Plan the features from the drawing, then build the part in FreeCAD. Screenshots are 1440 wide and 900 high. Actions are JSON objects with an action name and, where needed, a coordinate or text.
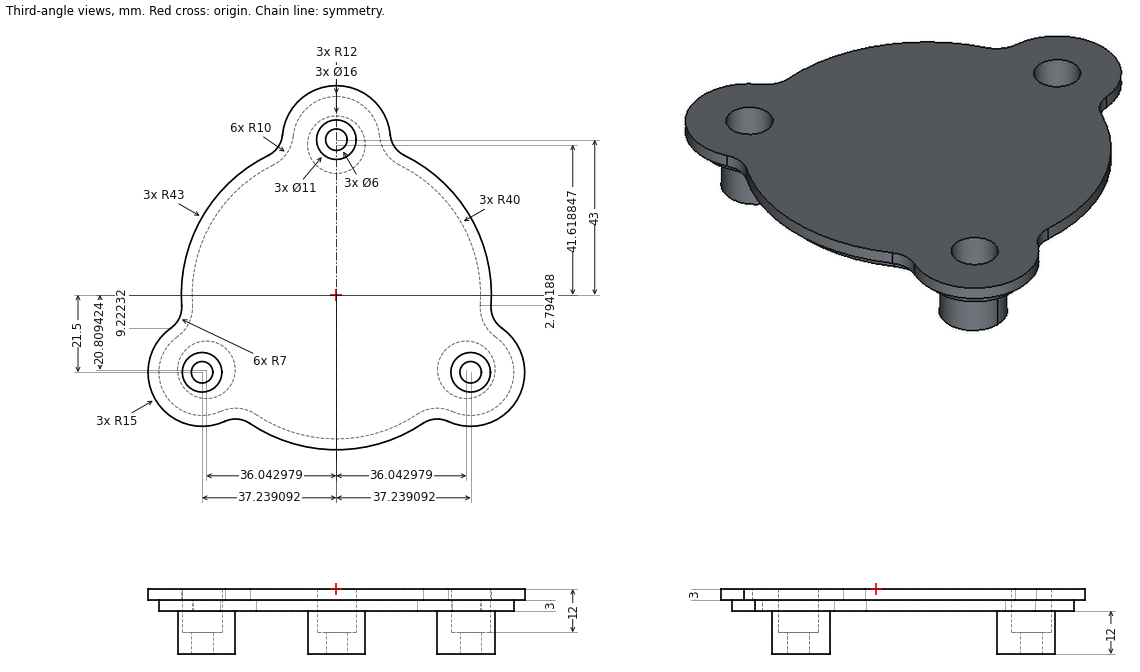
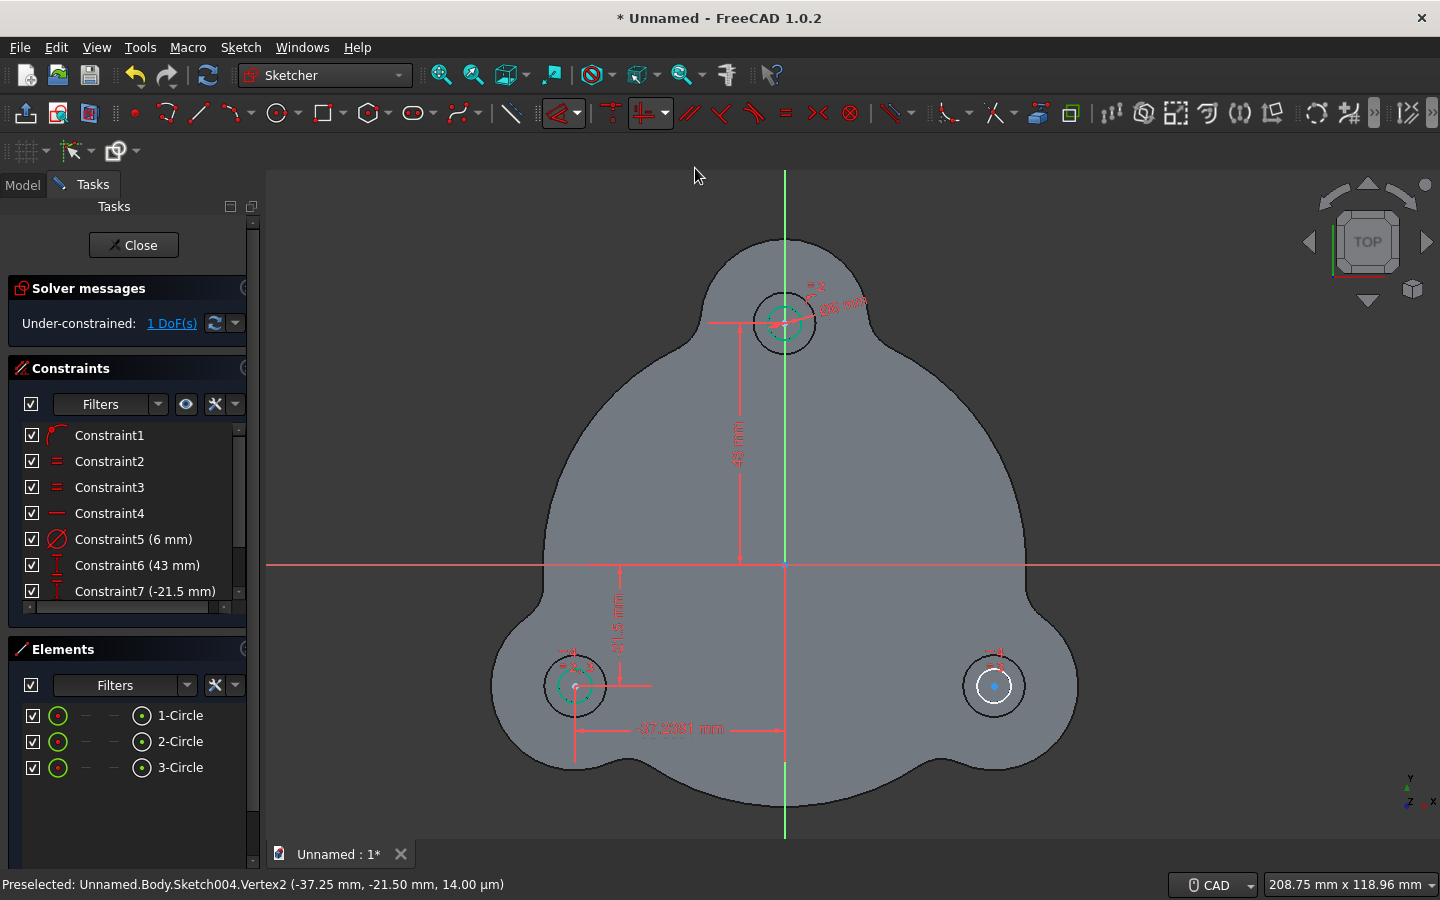
{"action": "left_click", "coordinate": [994, 686]}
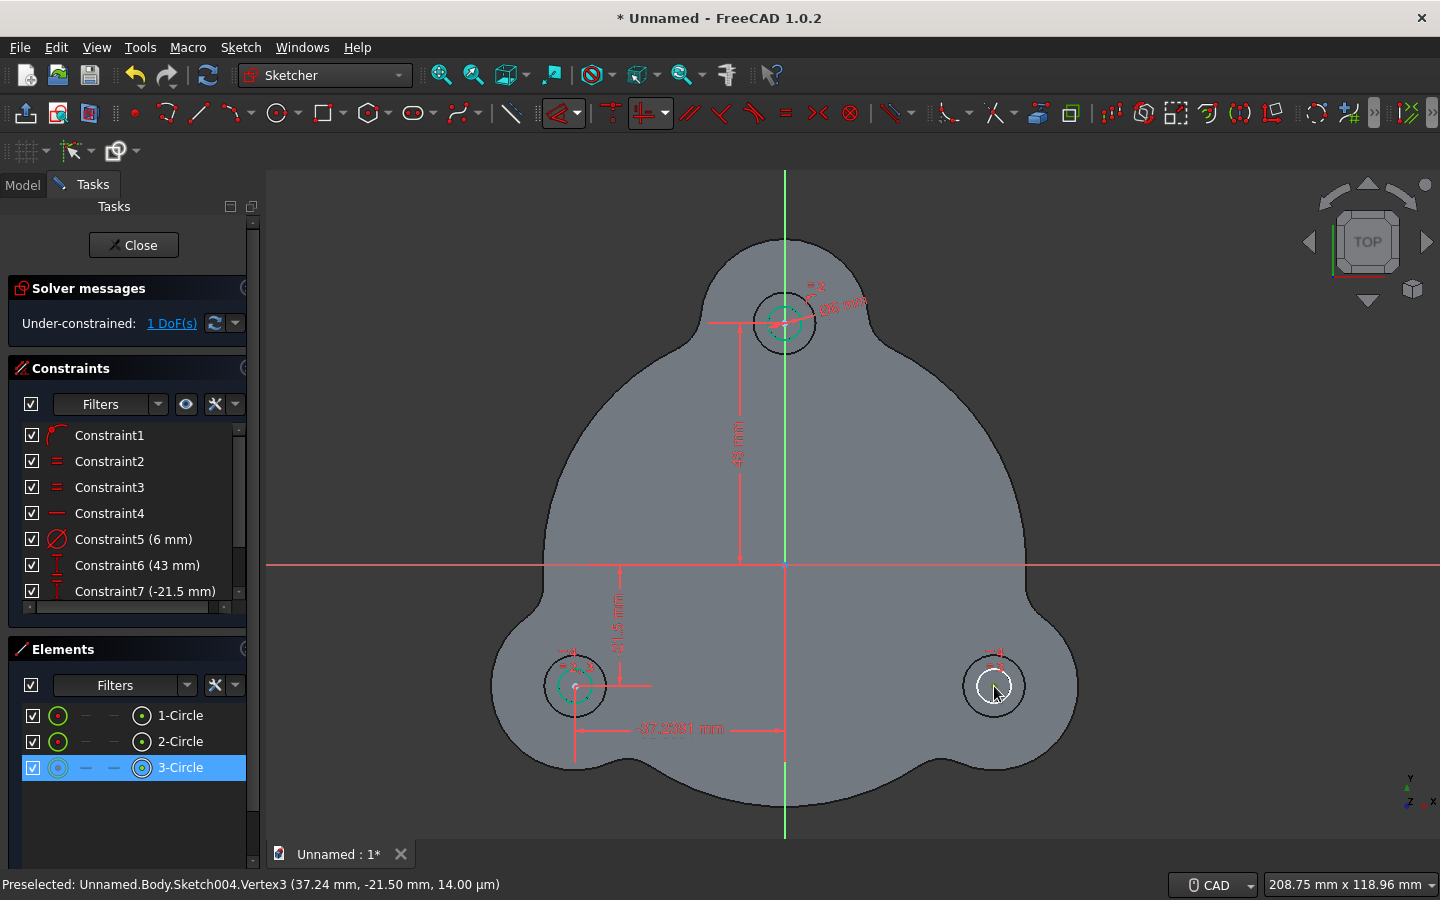
{"action": "key", "text": "l"}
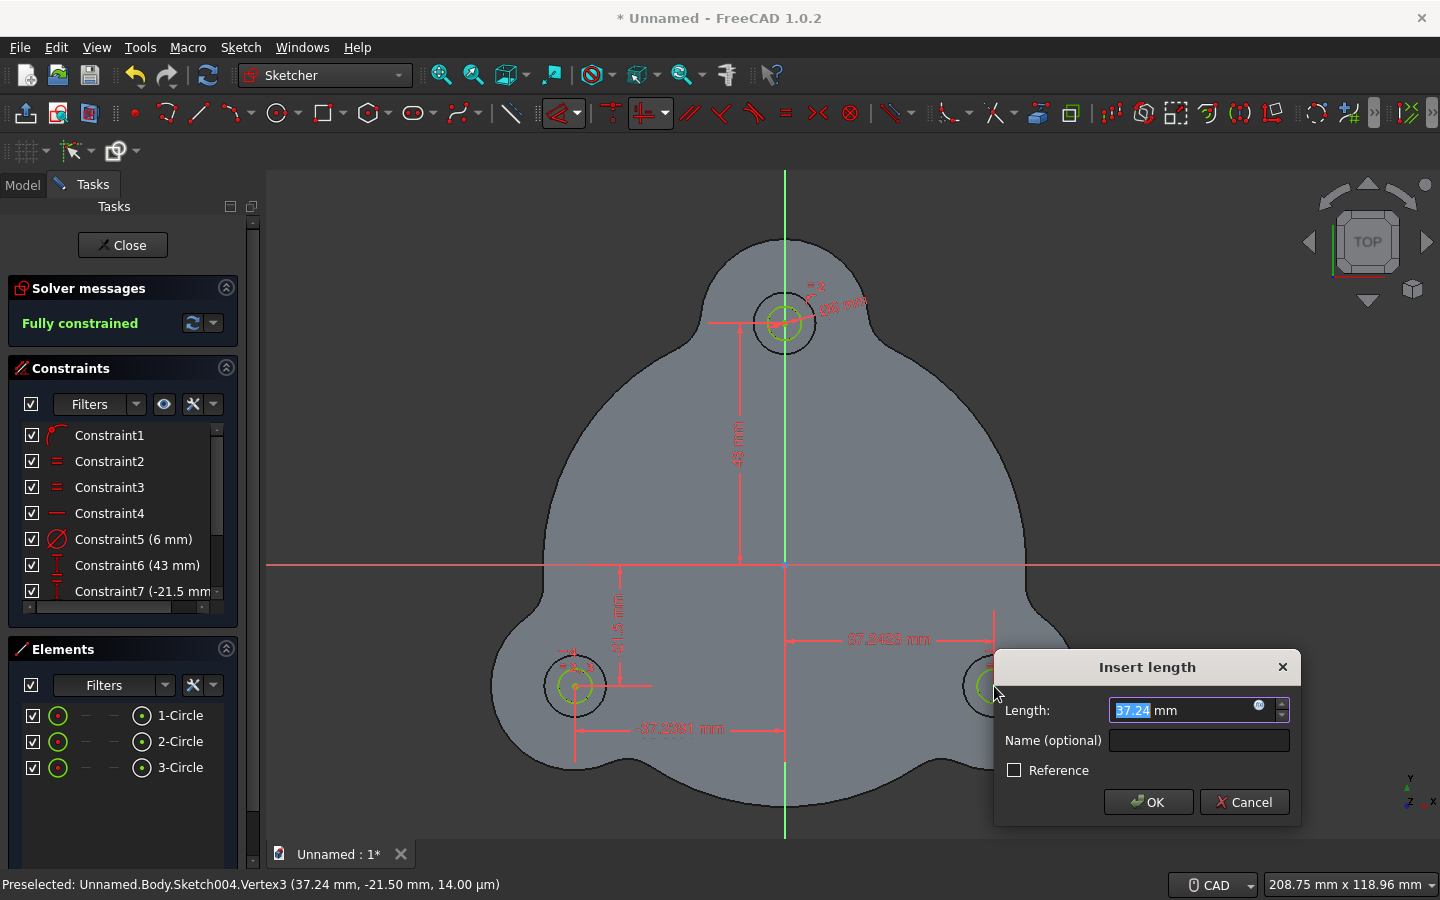
{"action": "type", "text": "37.239092"}
{"action": "key", "text": "Return"}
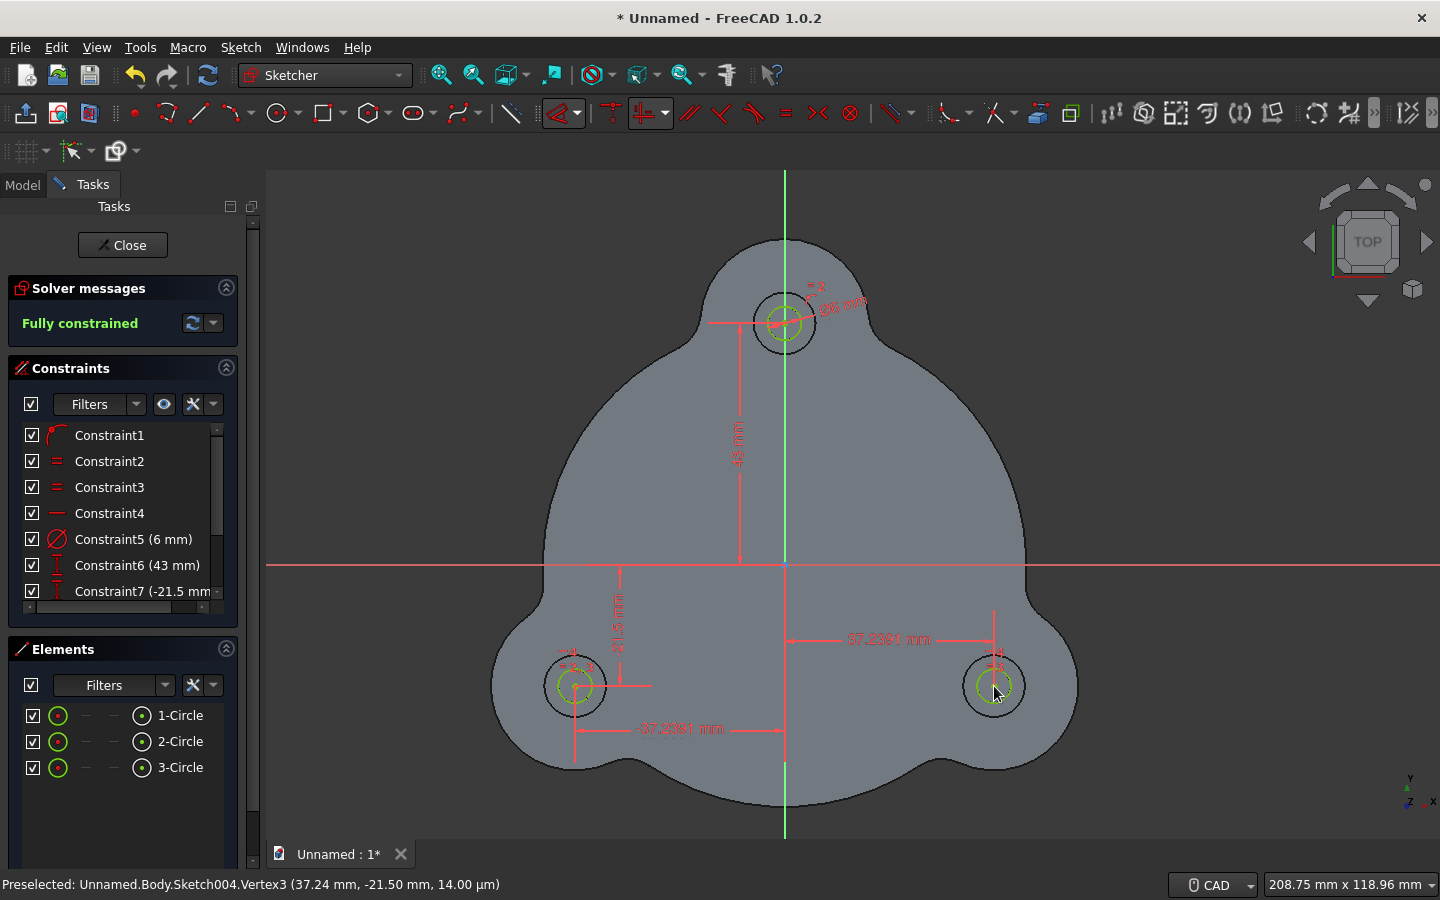
{"action": "left_click", "coordinate": [123, 245]}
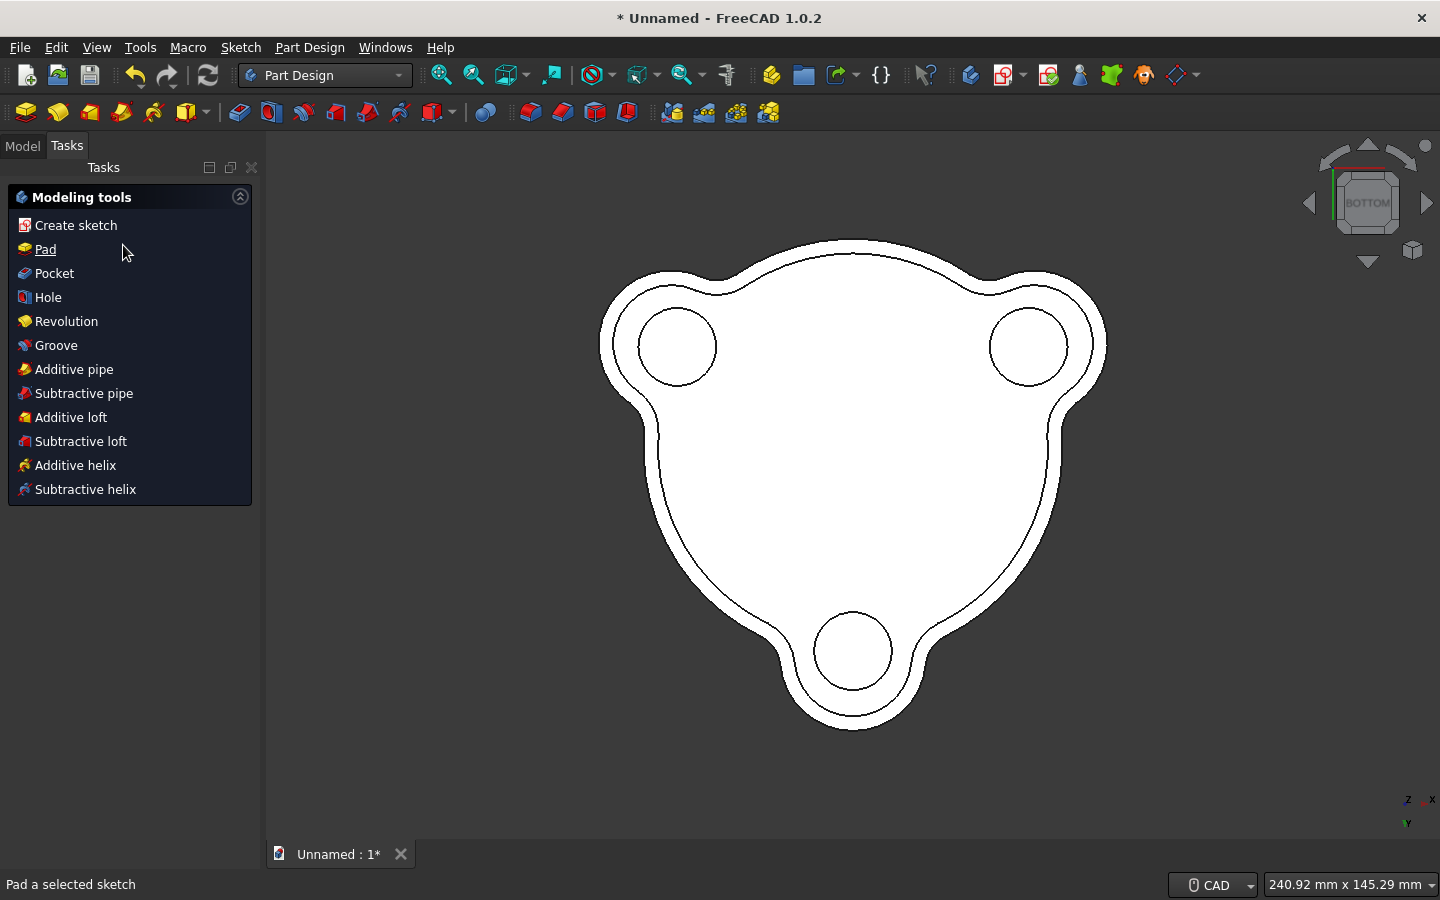
{"action": "left_click", "coordinate": [240, 112]}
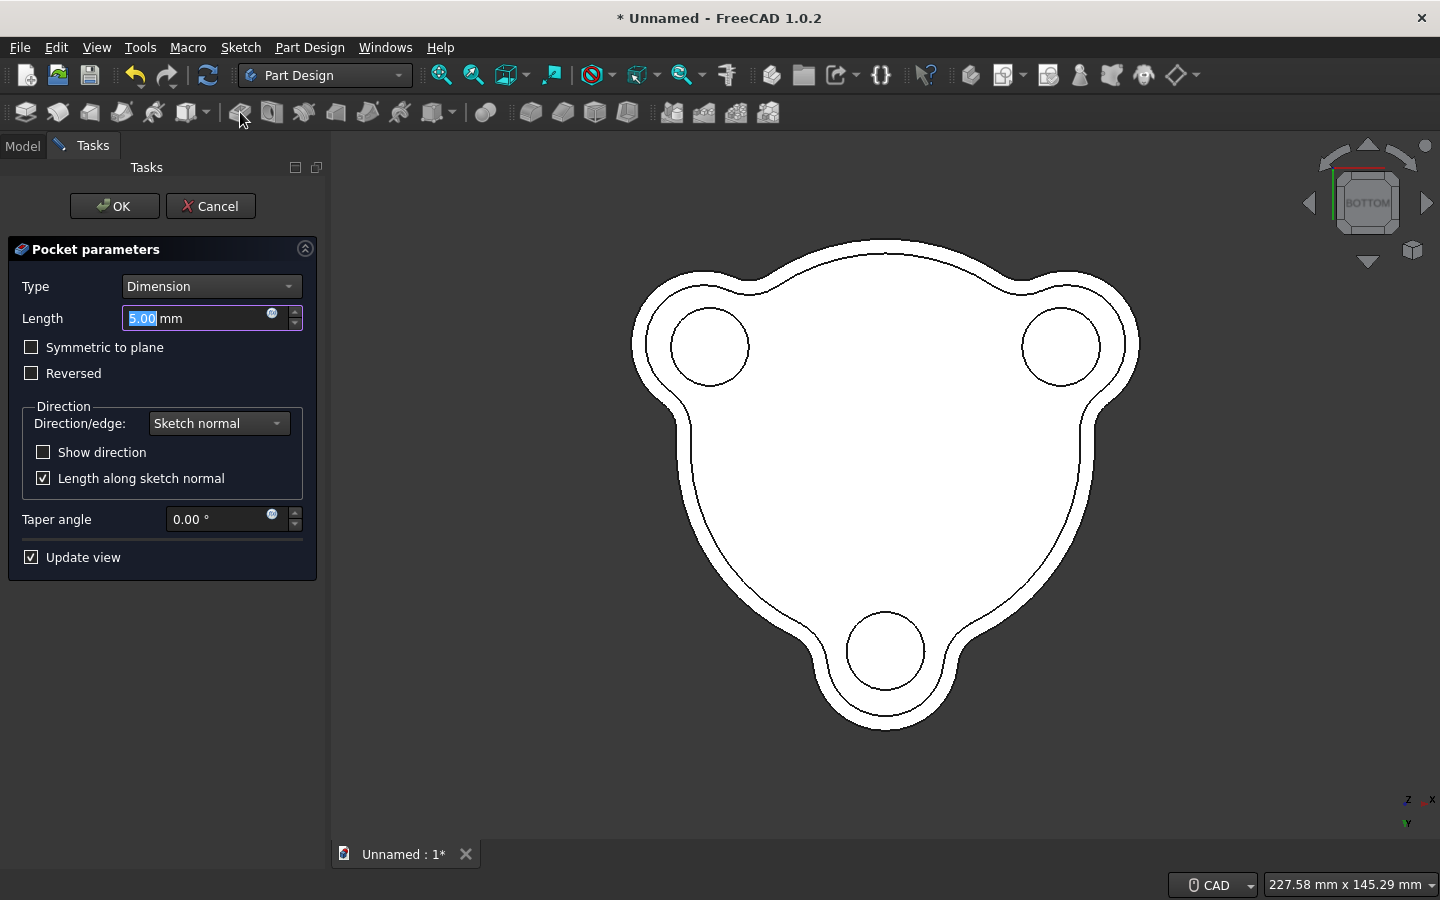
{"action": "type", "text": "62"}
{"action": "key", "text": "Tab"}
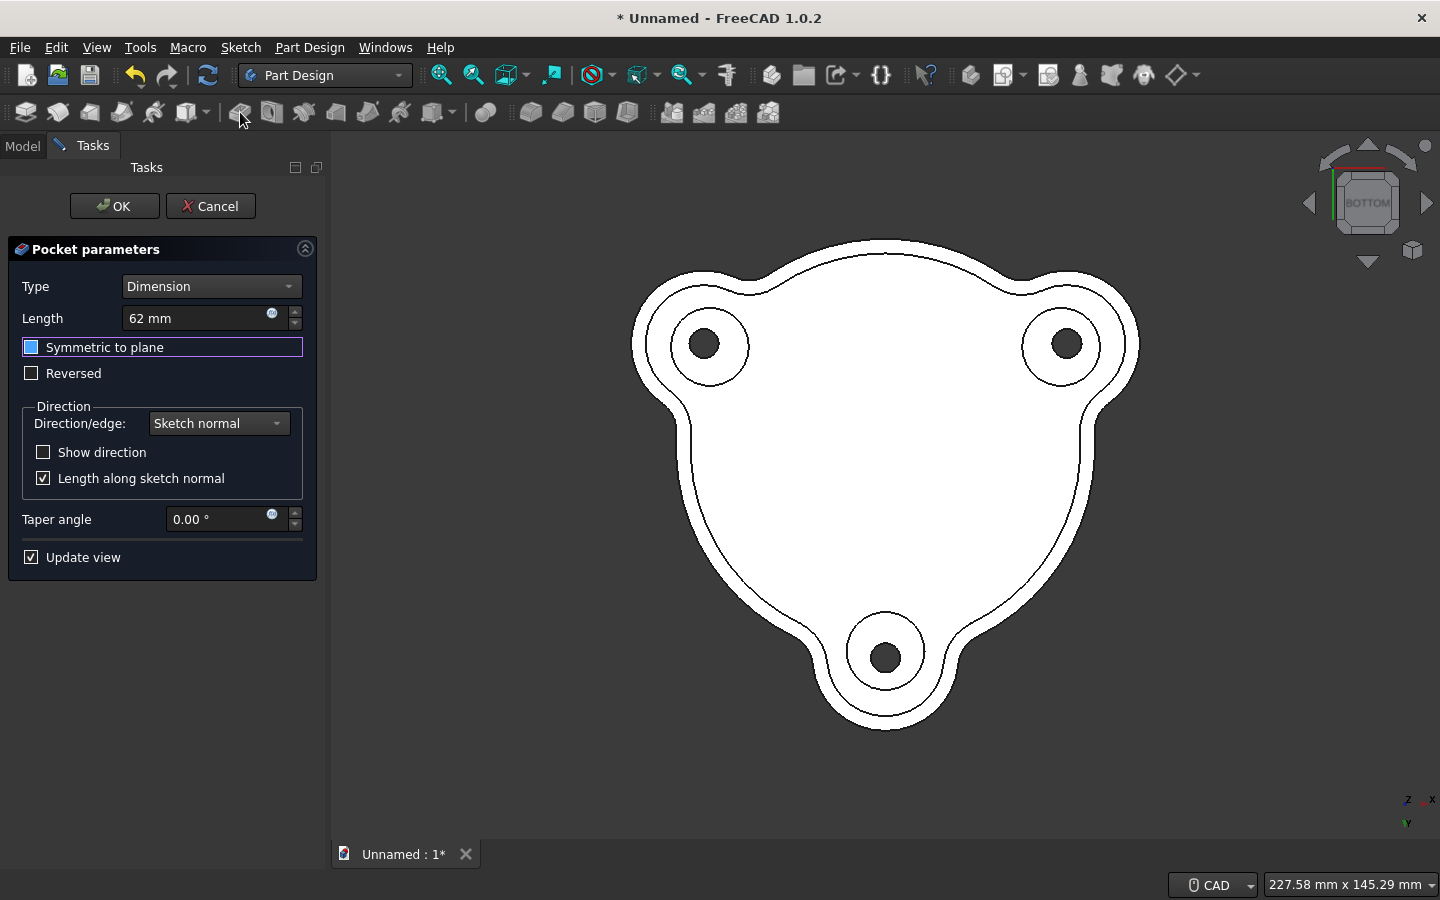
{"action": "left_click", "coordinate": [115, 206]}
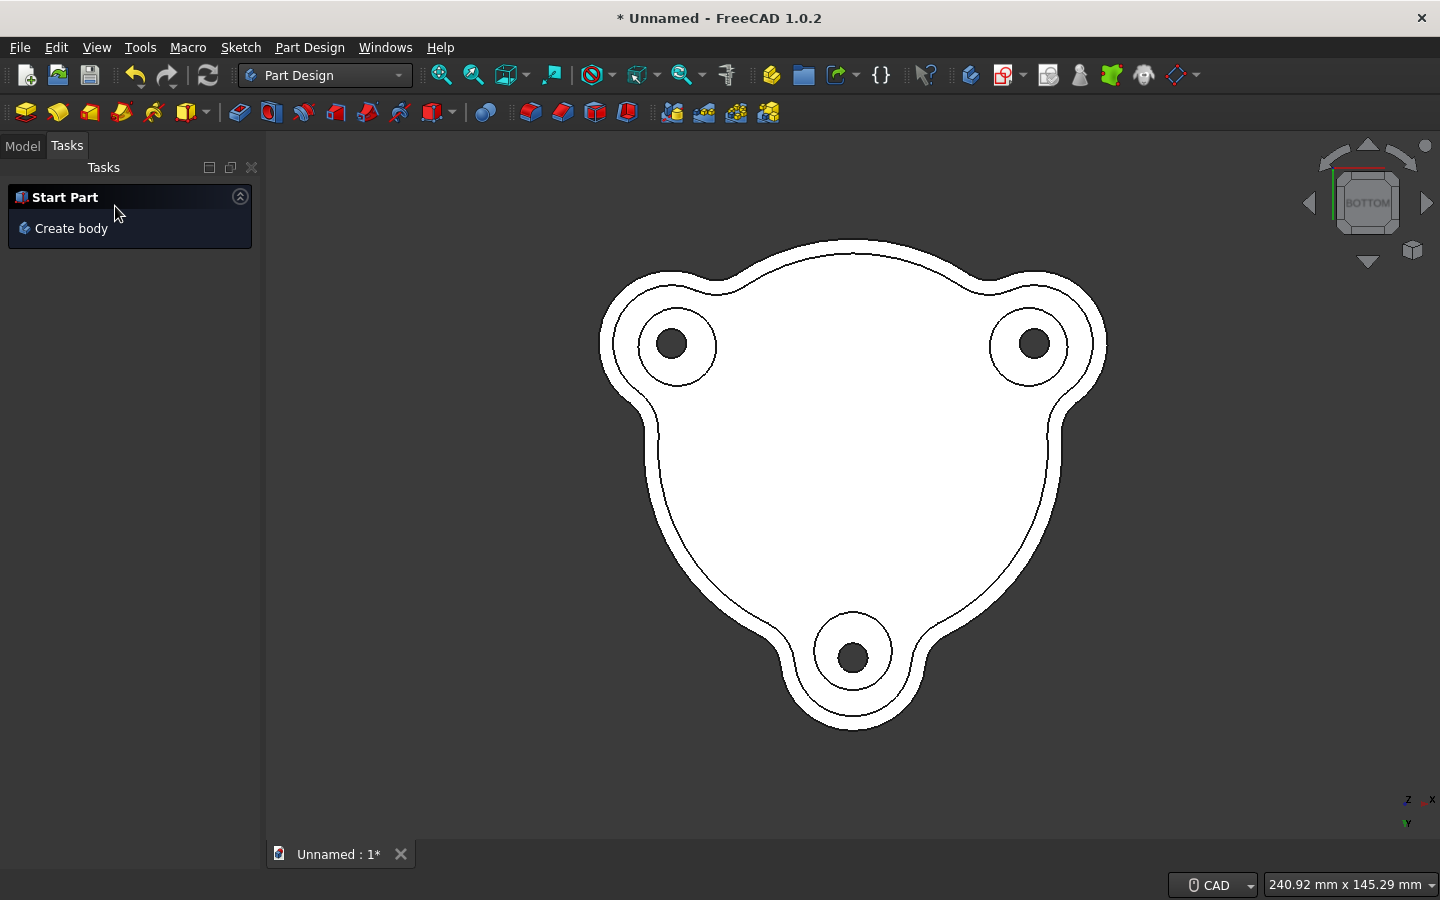
{"action": "key", "text": "0"}